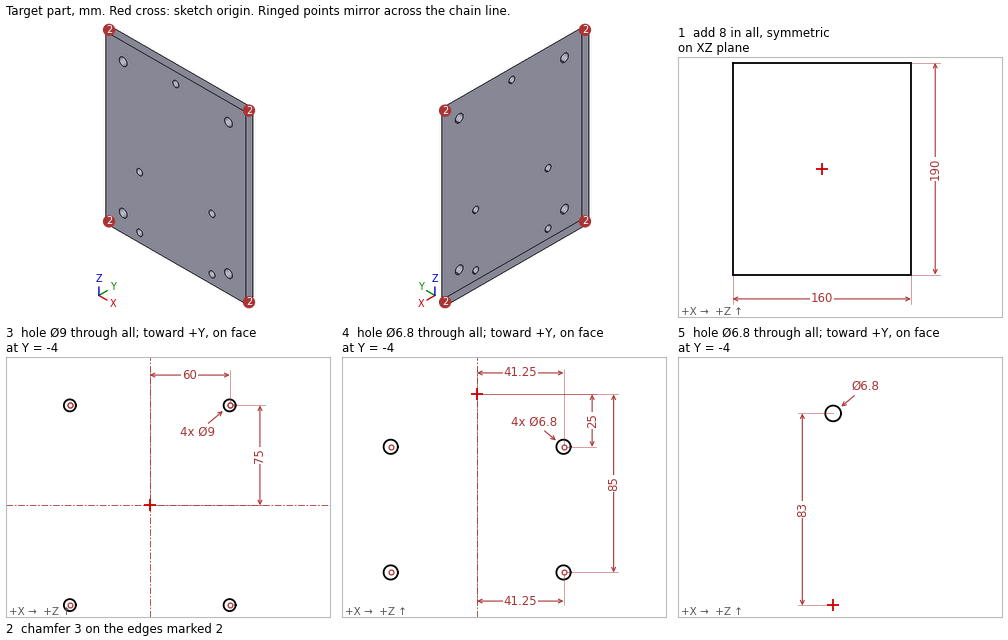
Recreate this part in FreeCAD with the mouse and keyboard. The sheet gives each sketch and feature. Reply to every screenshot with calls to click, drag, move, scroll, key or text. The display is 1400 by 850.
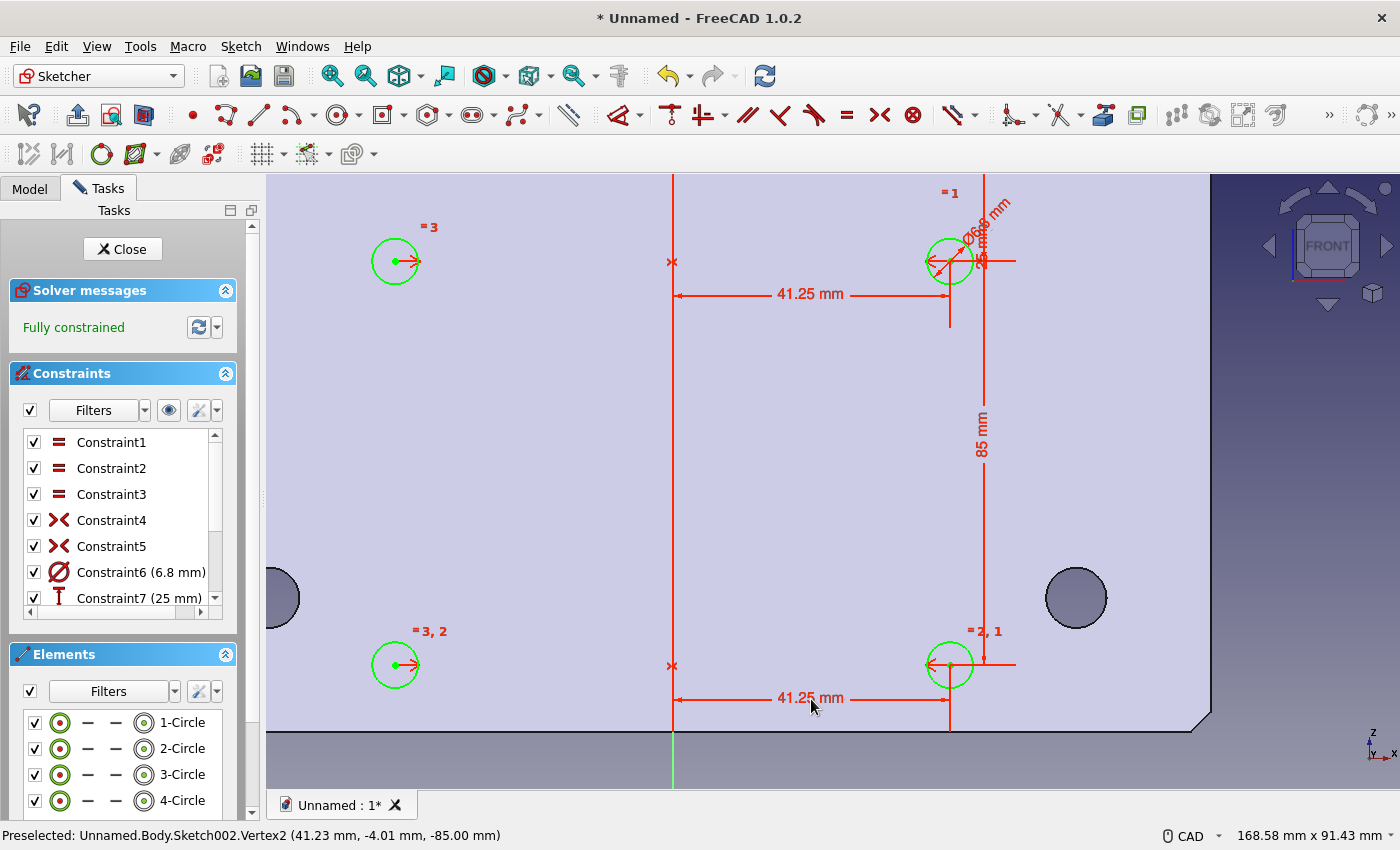
click(123, 249)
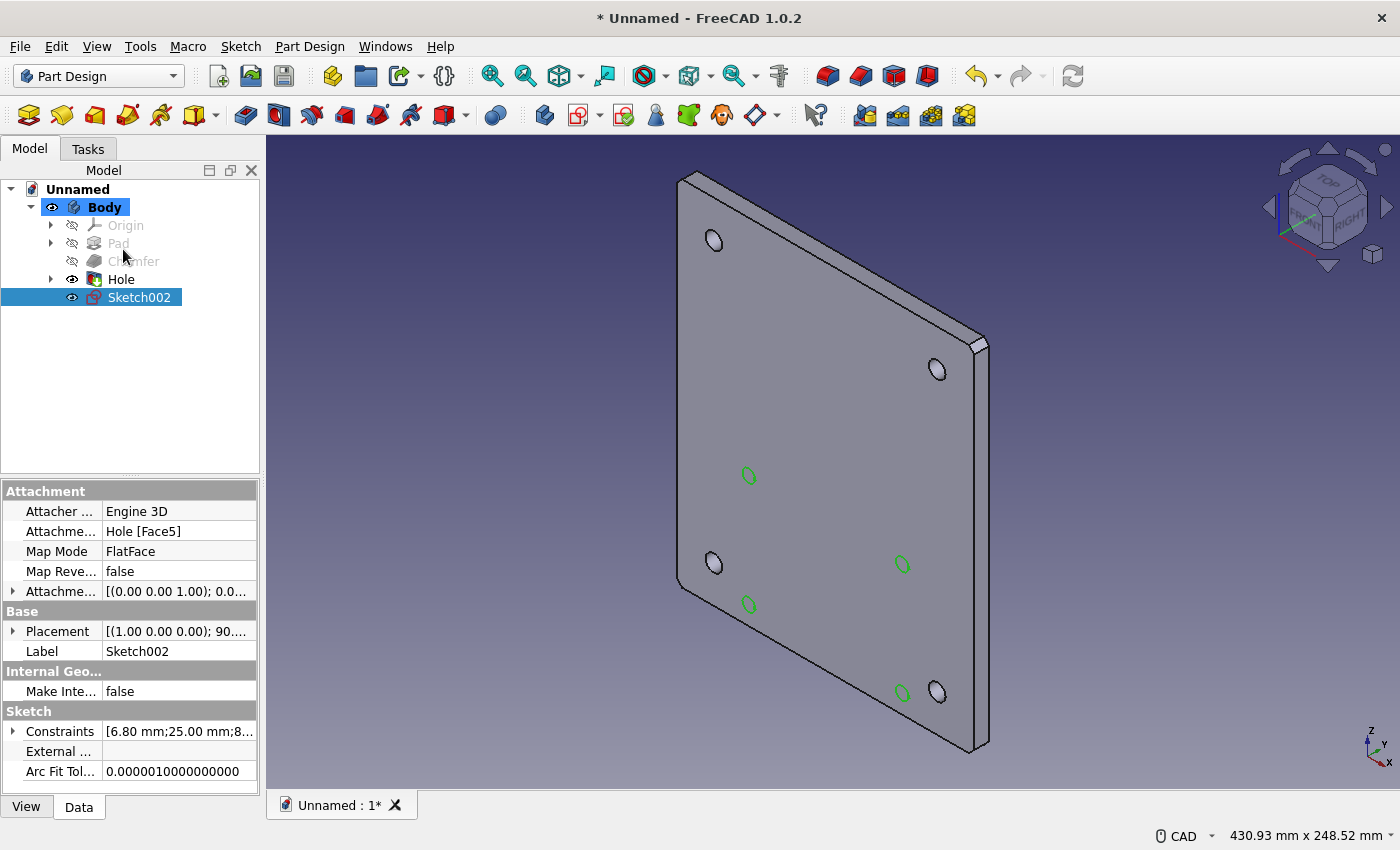
click(279, 116)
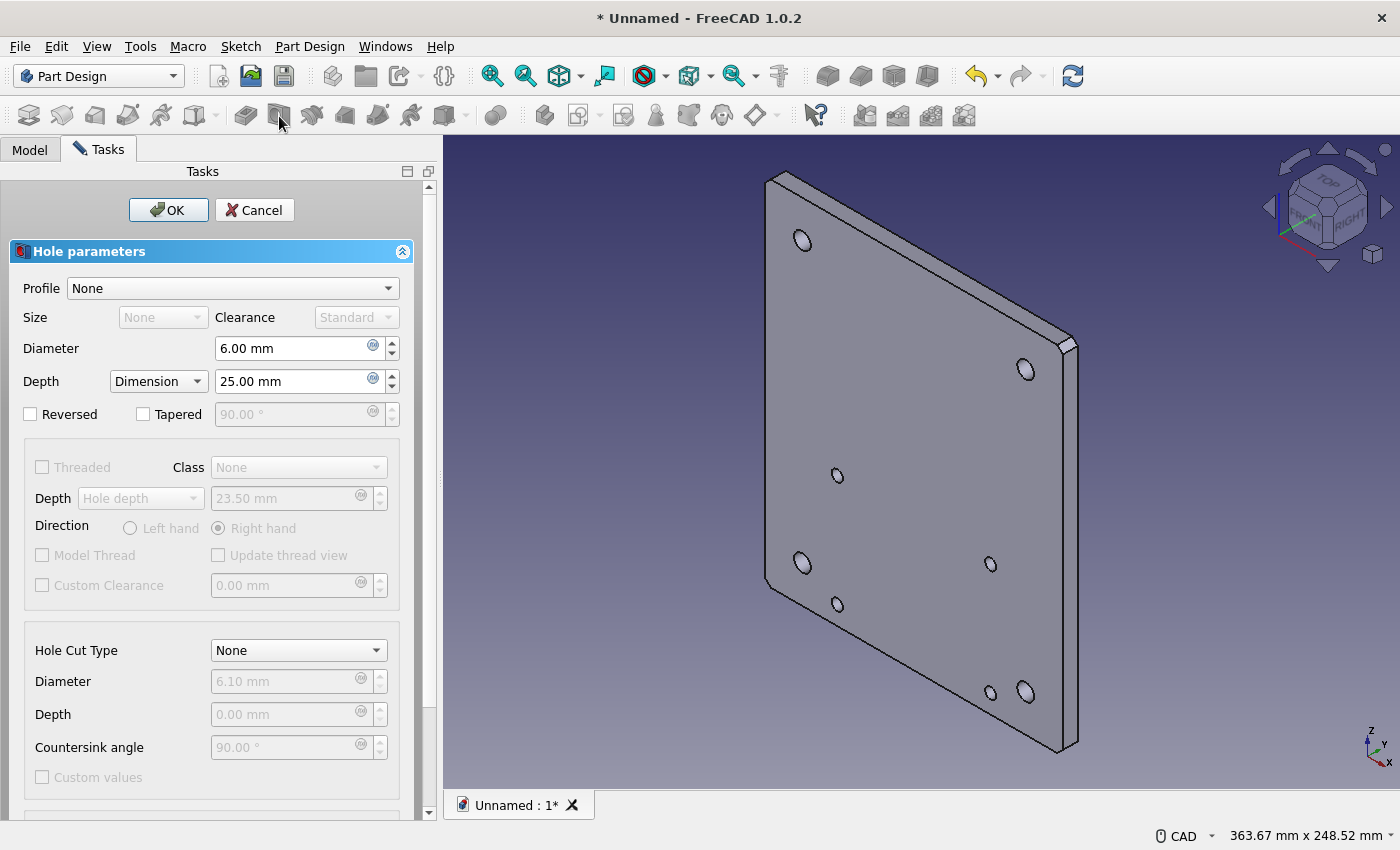
triple_click(300, 348)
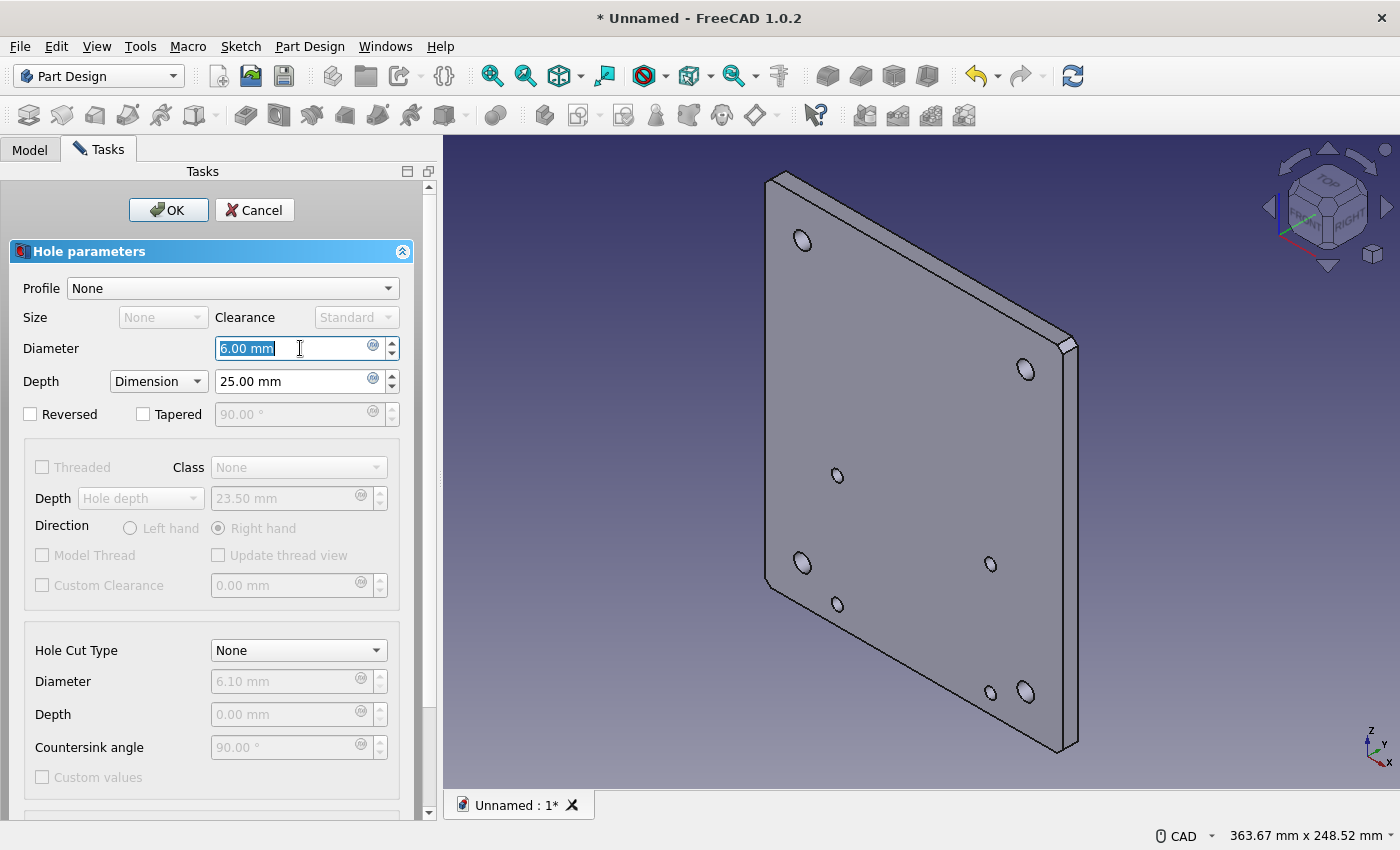
text(6.8)
key(Tab)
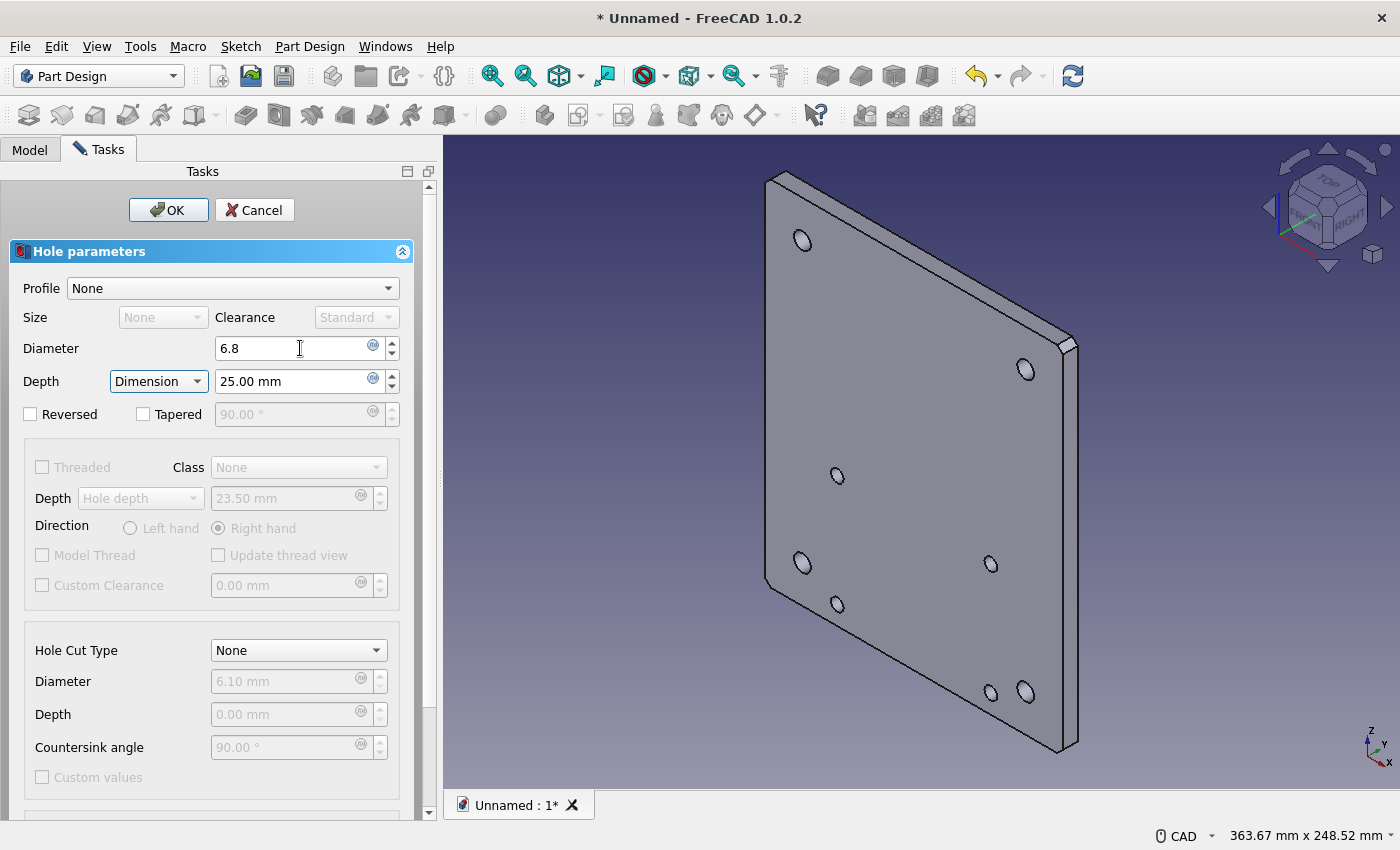
click(160, 382)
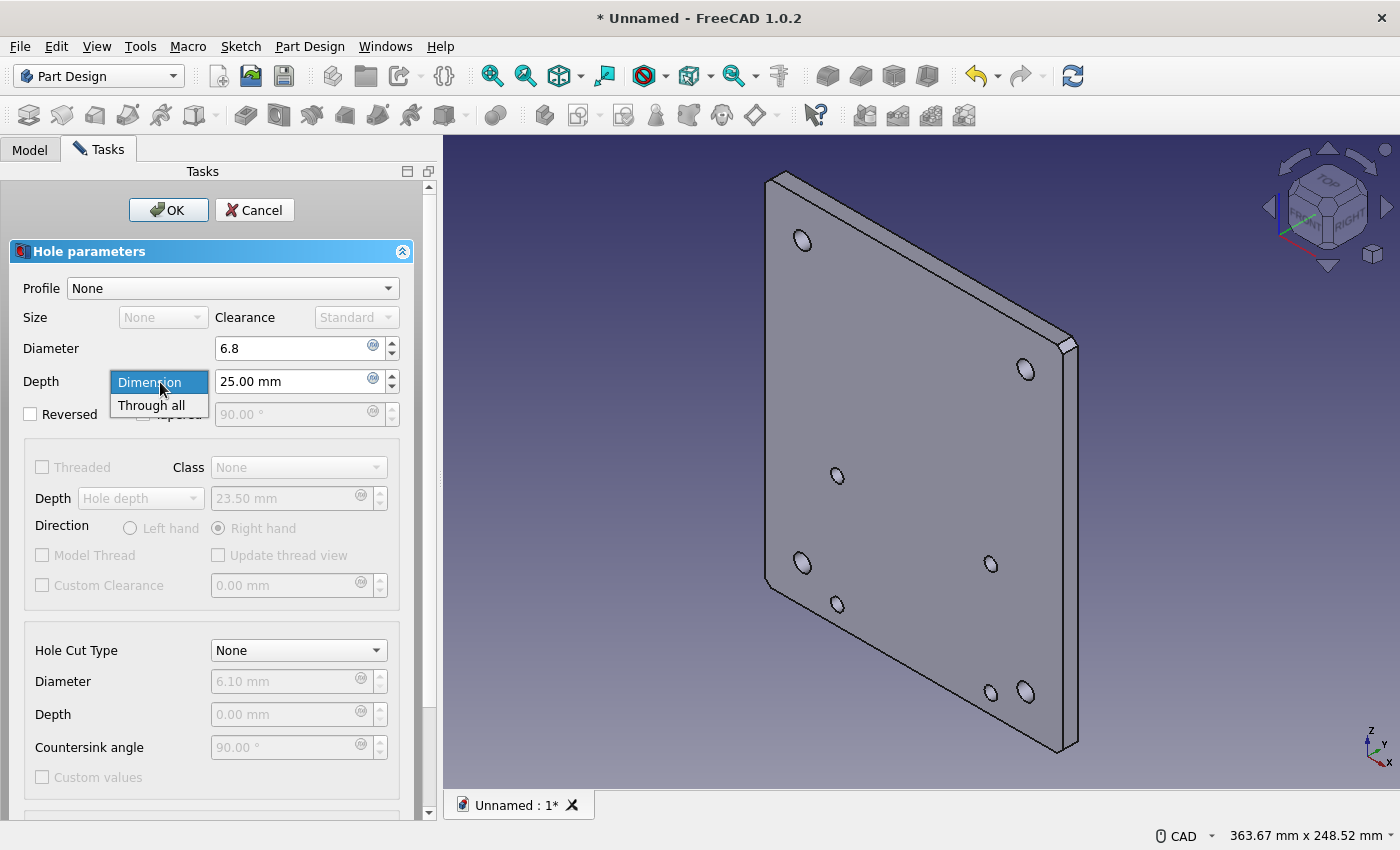
click(158, 406)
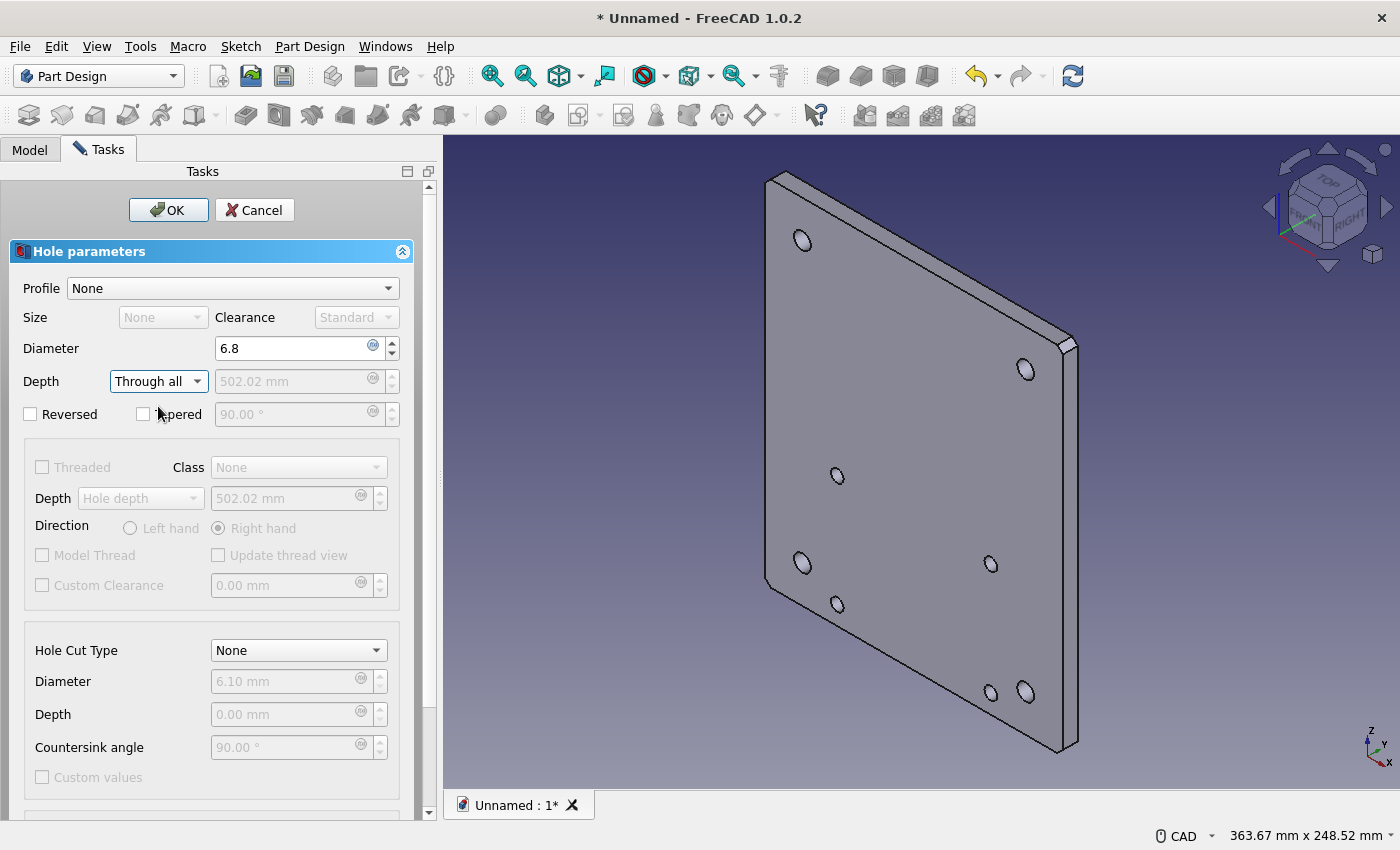
click(169, 210)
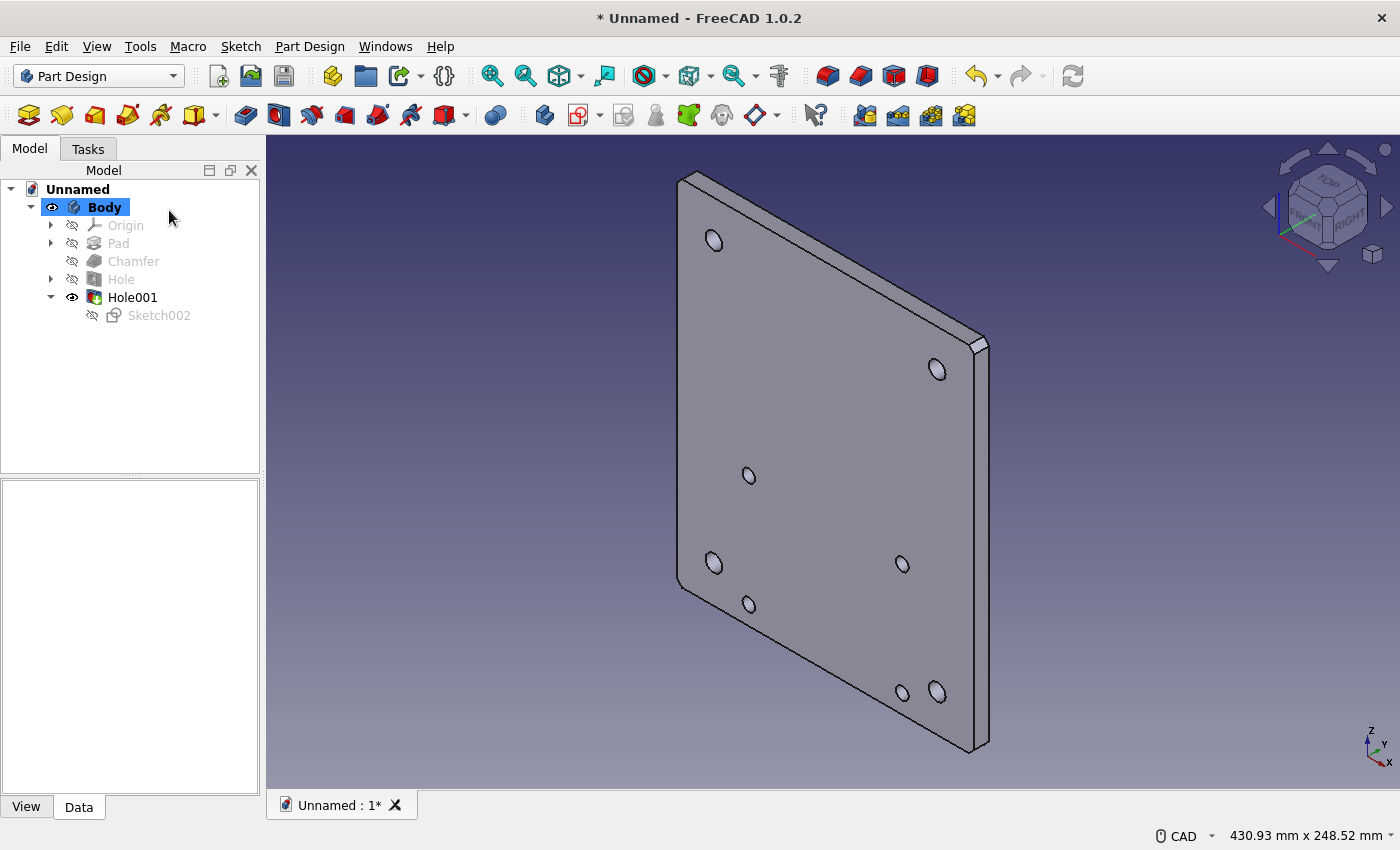
click(826, 407)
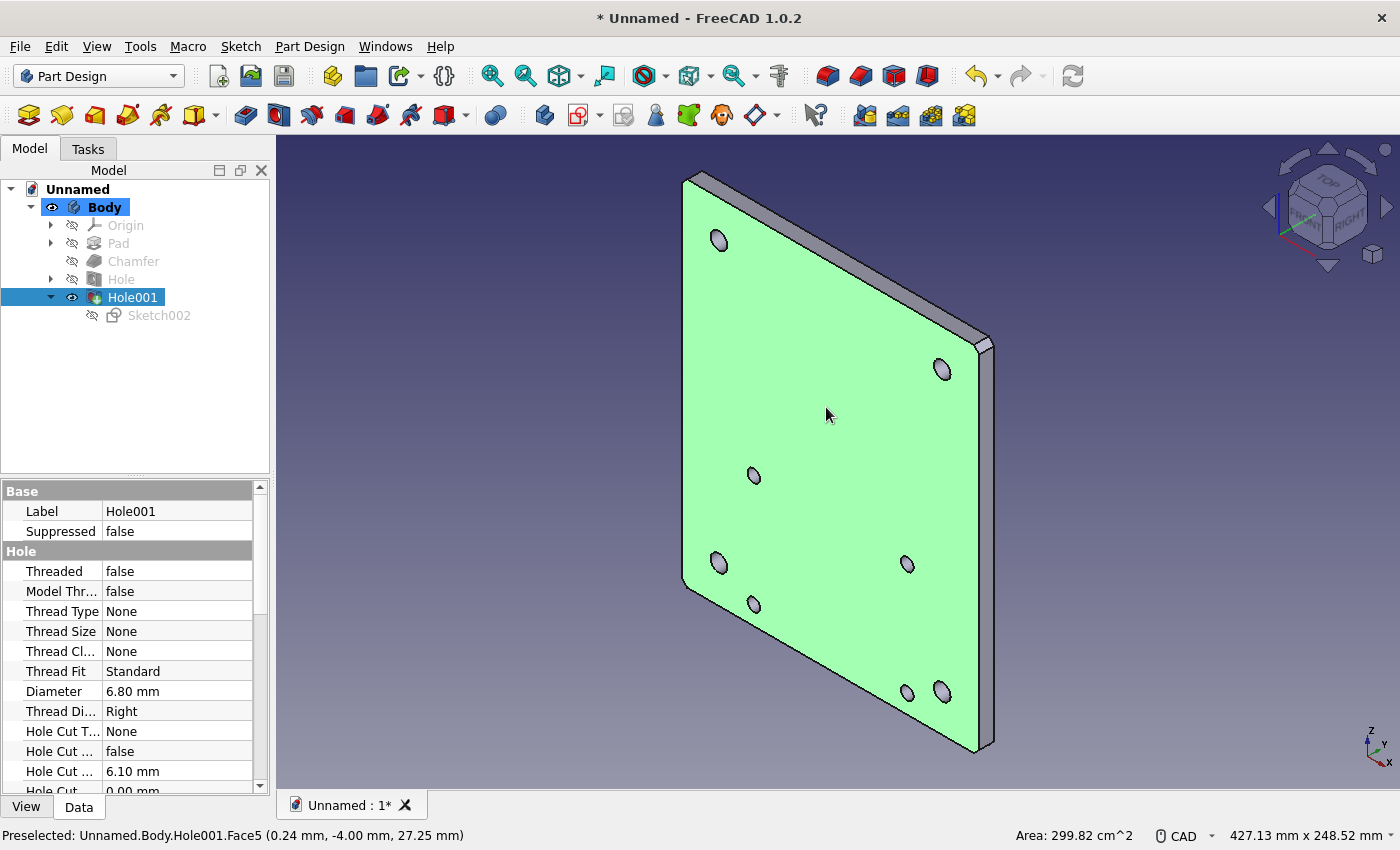
click(578, 116)